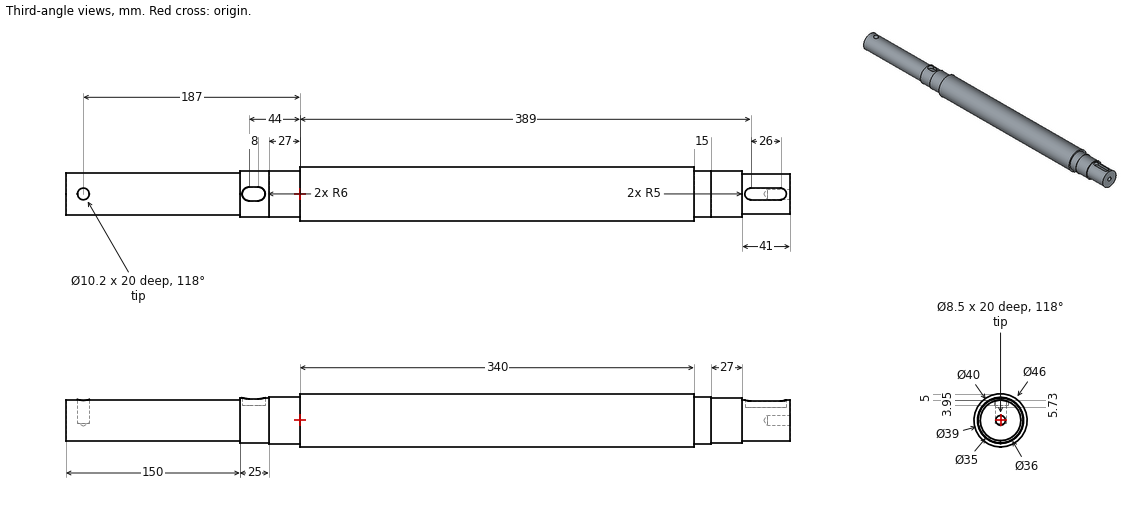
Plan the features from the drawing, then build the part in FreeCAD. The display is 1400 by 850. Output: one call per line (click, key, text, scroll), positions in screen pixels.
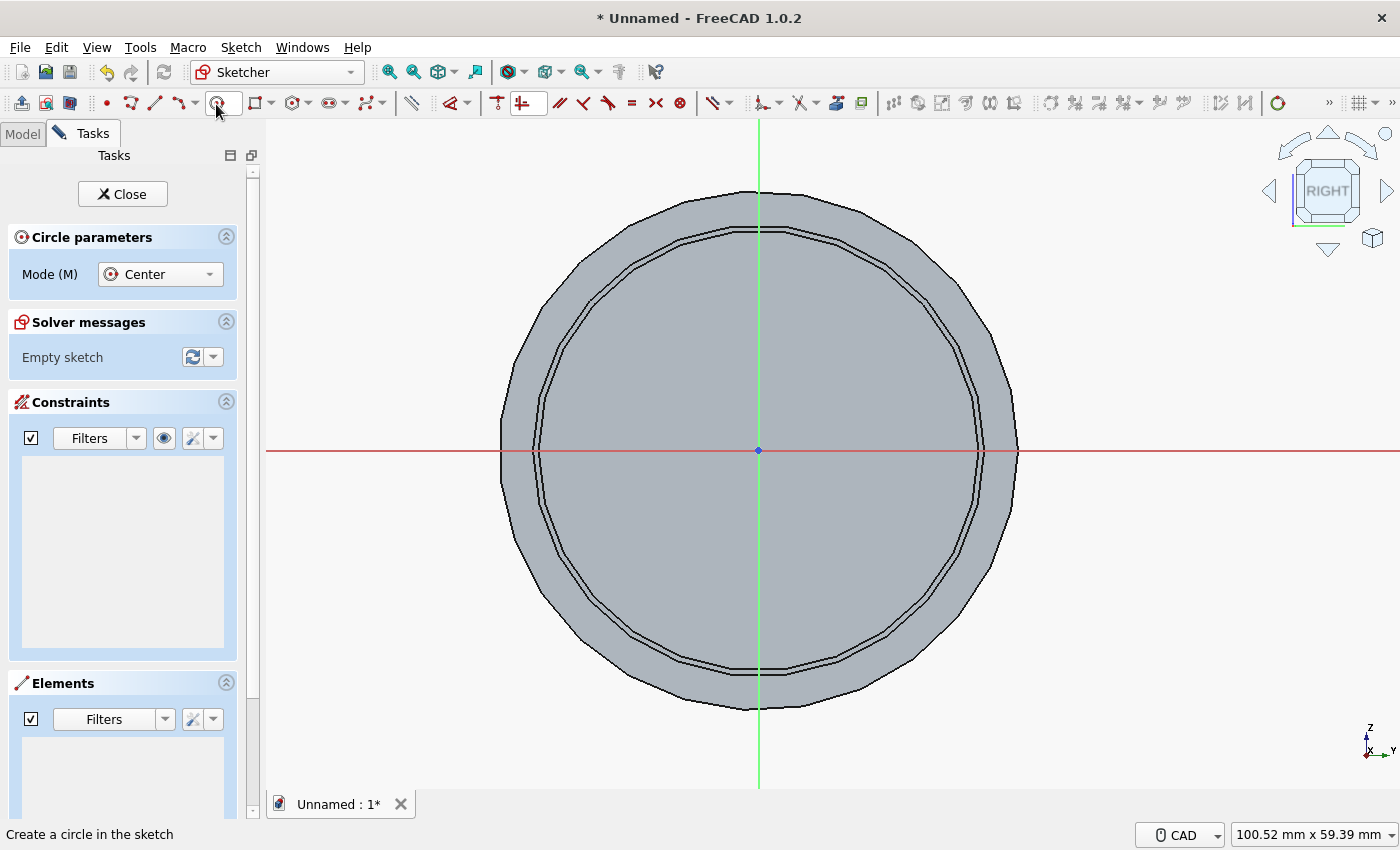
click(759, 451)
click(898, 311)
key(Escape)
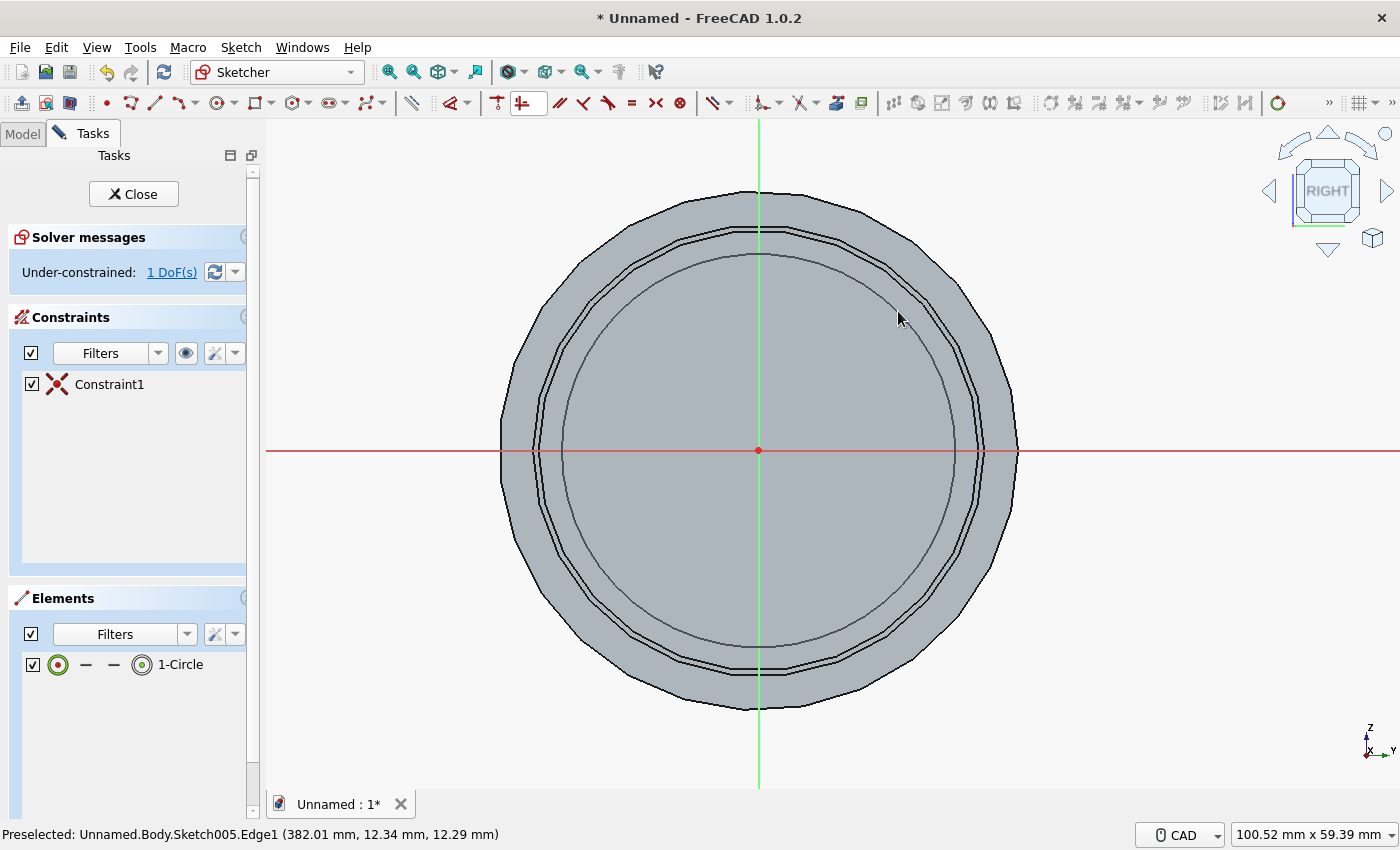
click(450, 104)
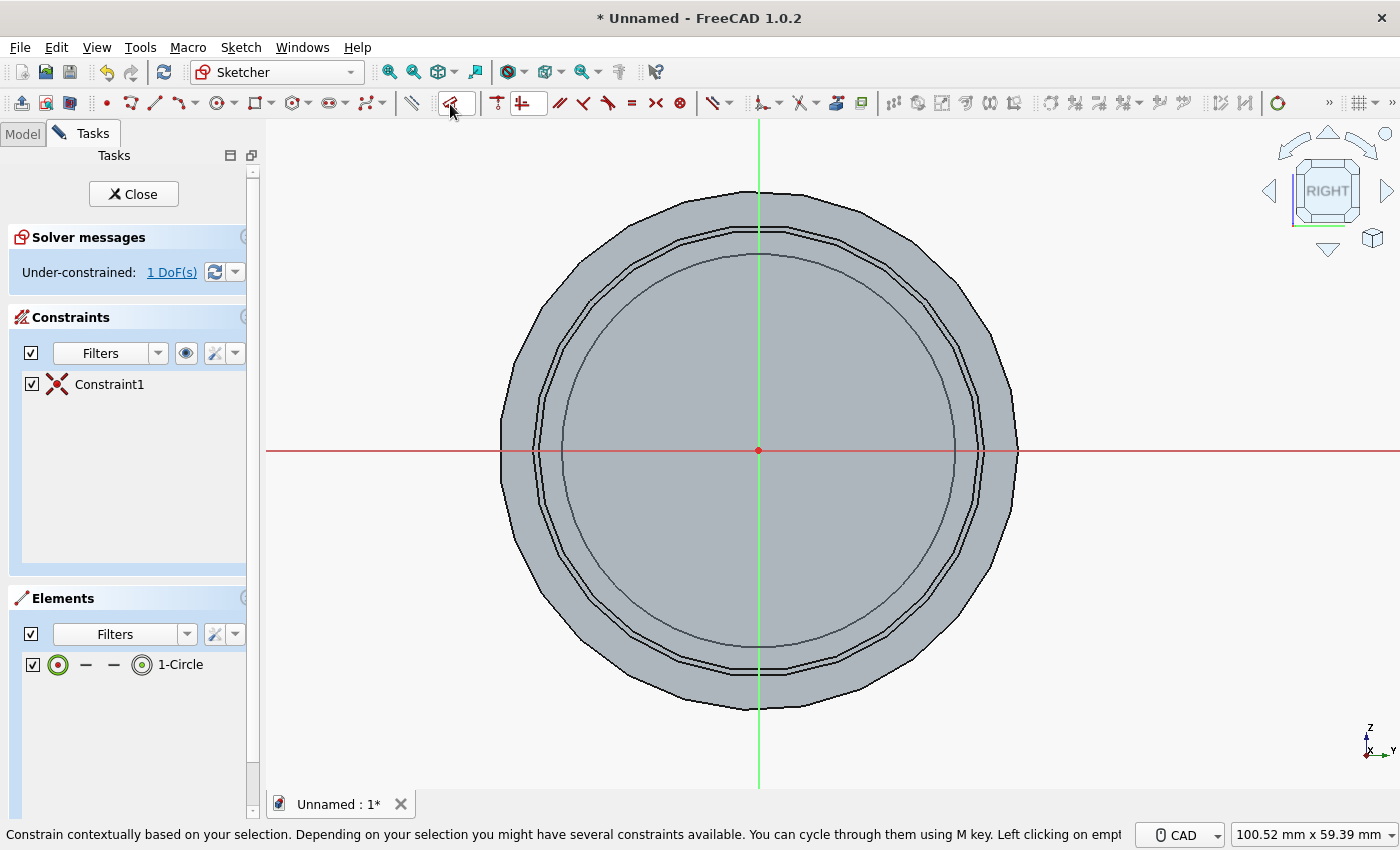
click(897, 311)
click(920, 288)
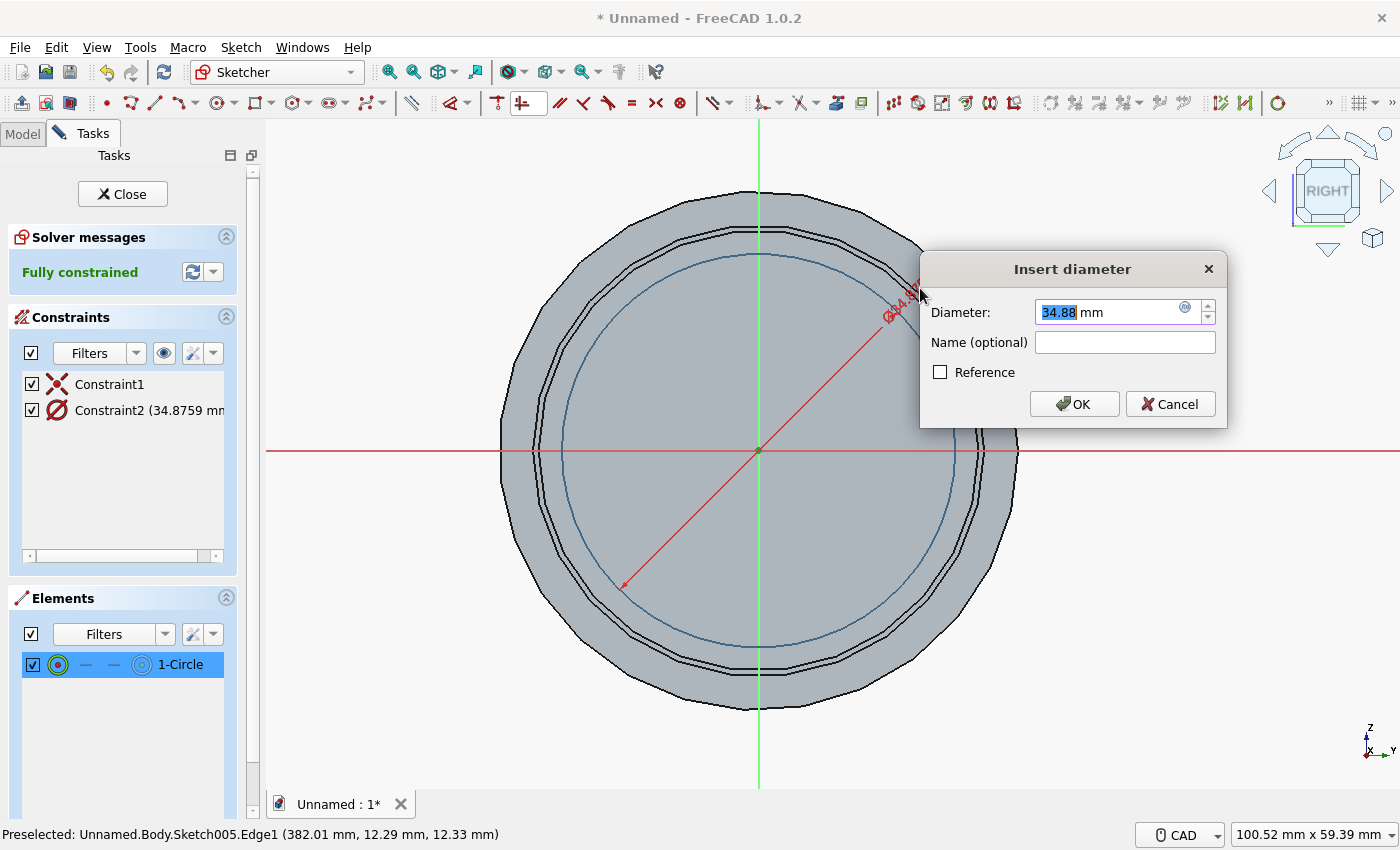
text(35)
key(Return)
key(Escape)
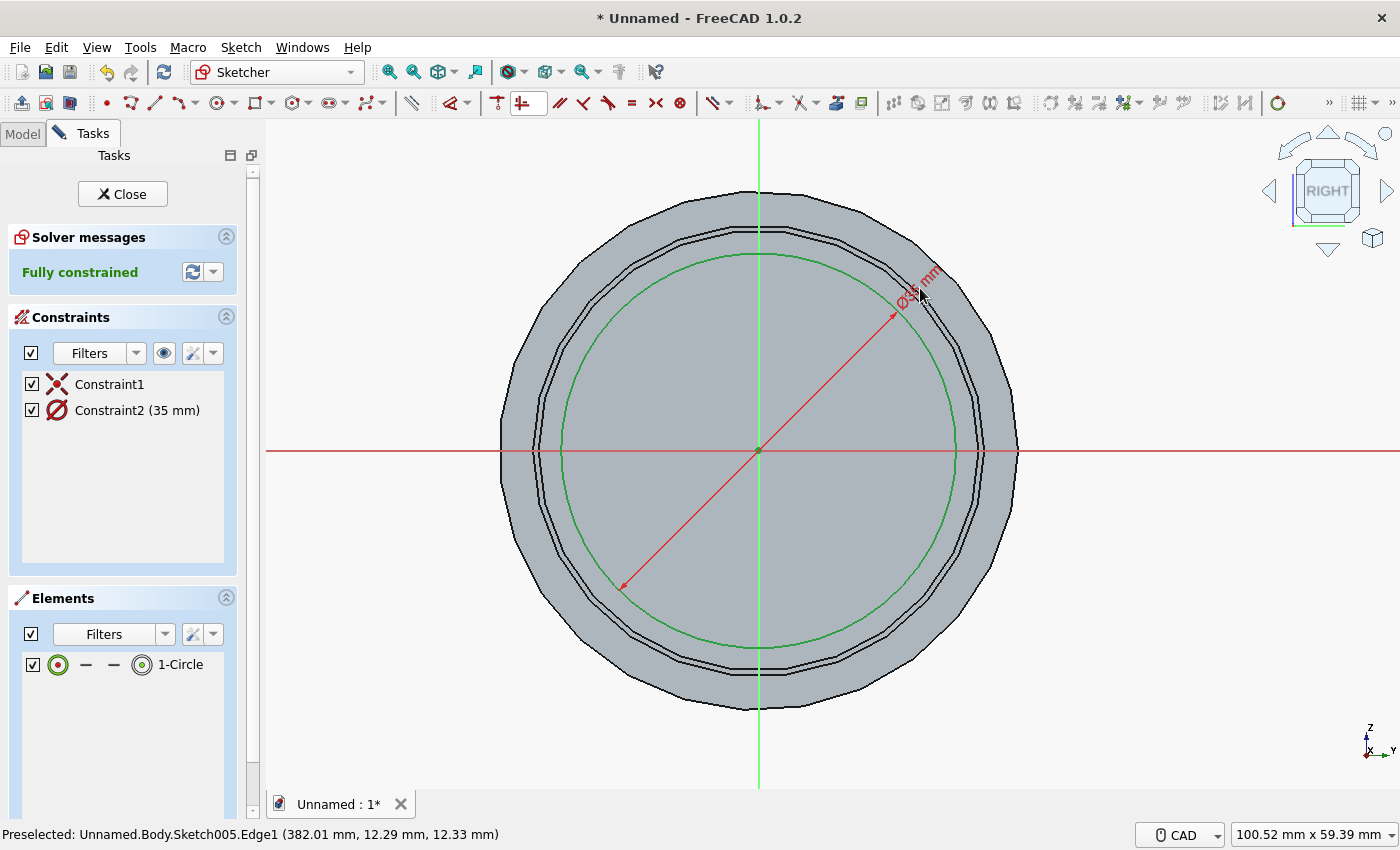
click(123, 194)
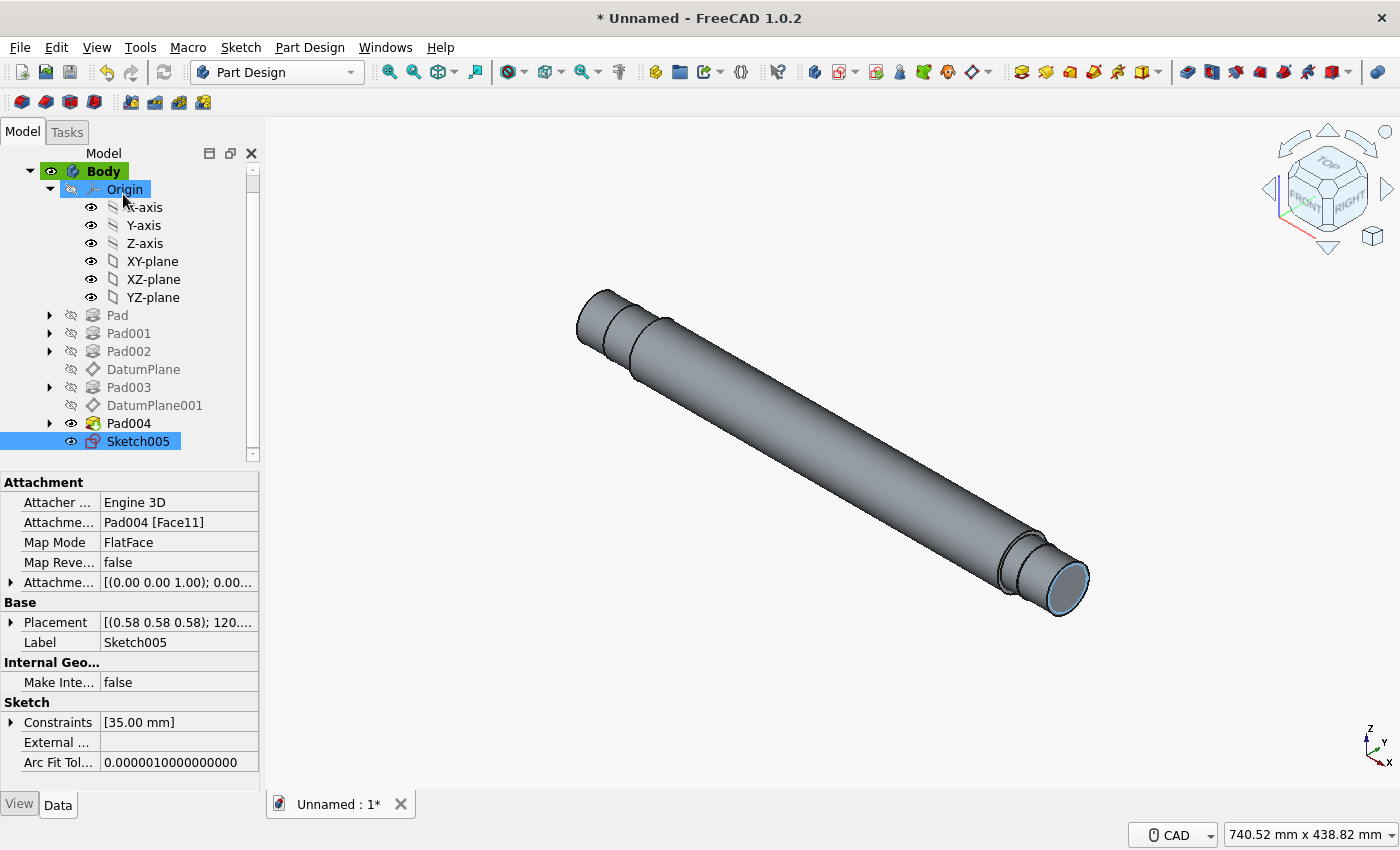
click(1022, 72)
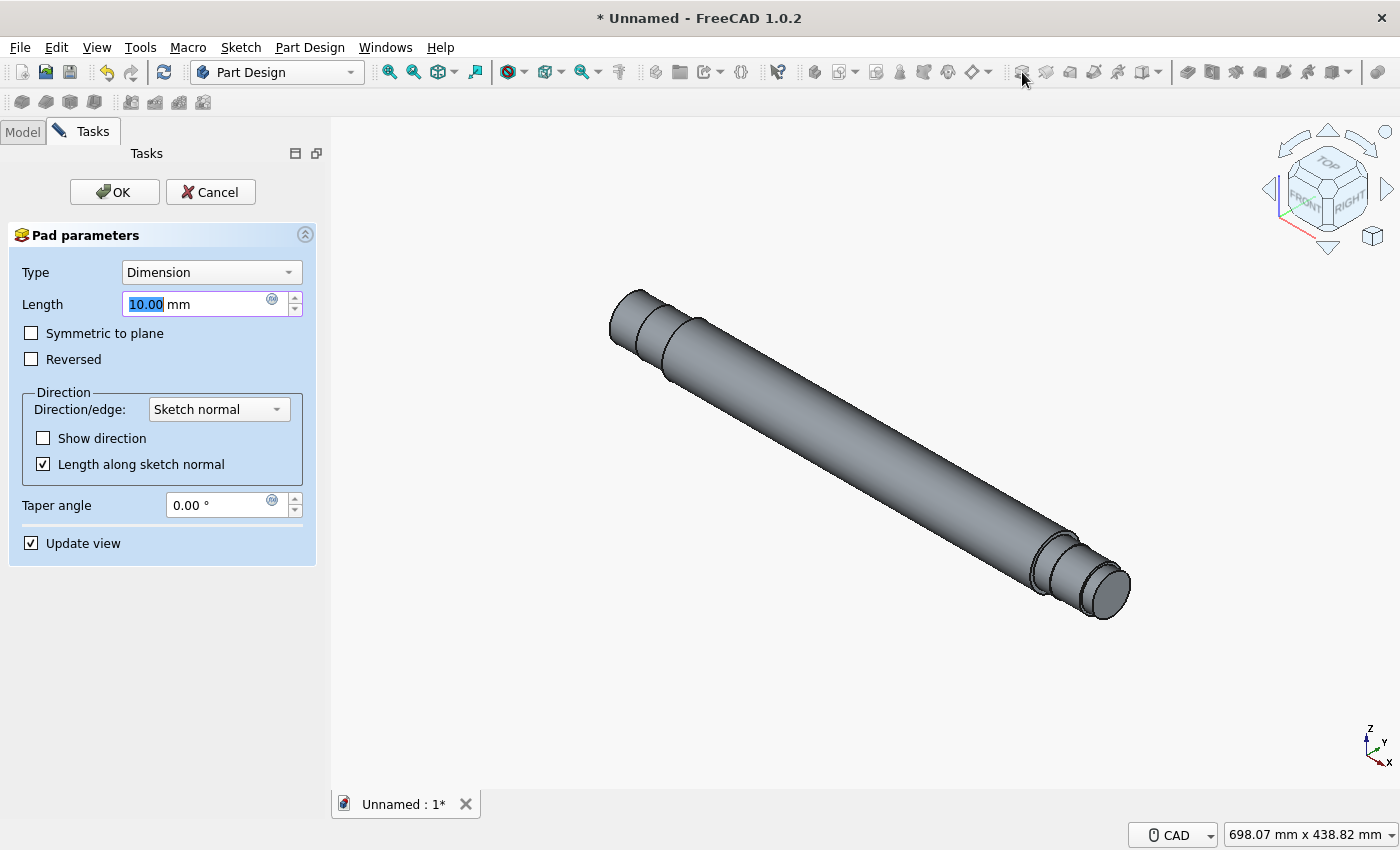
text(41)
key(Tab)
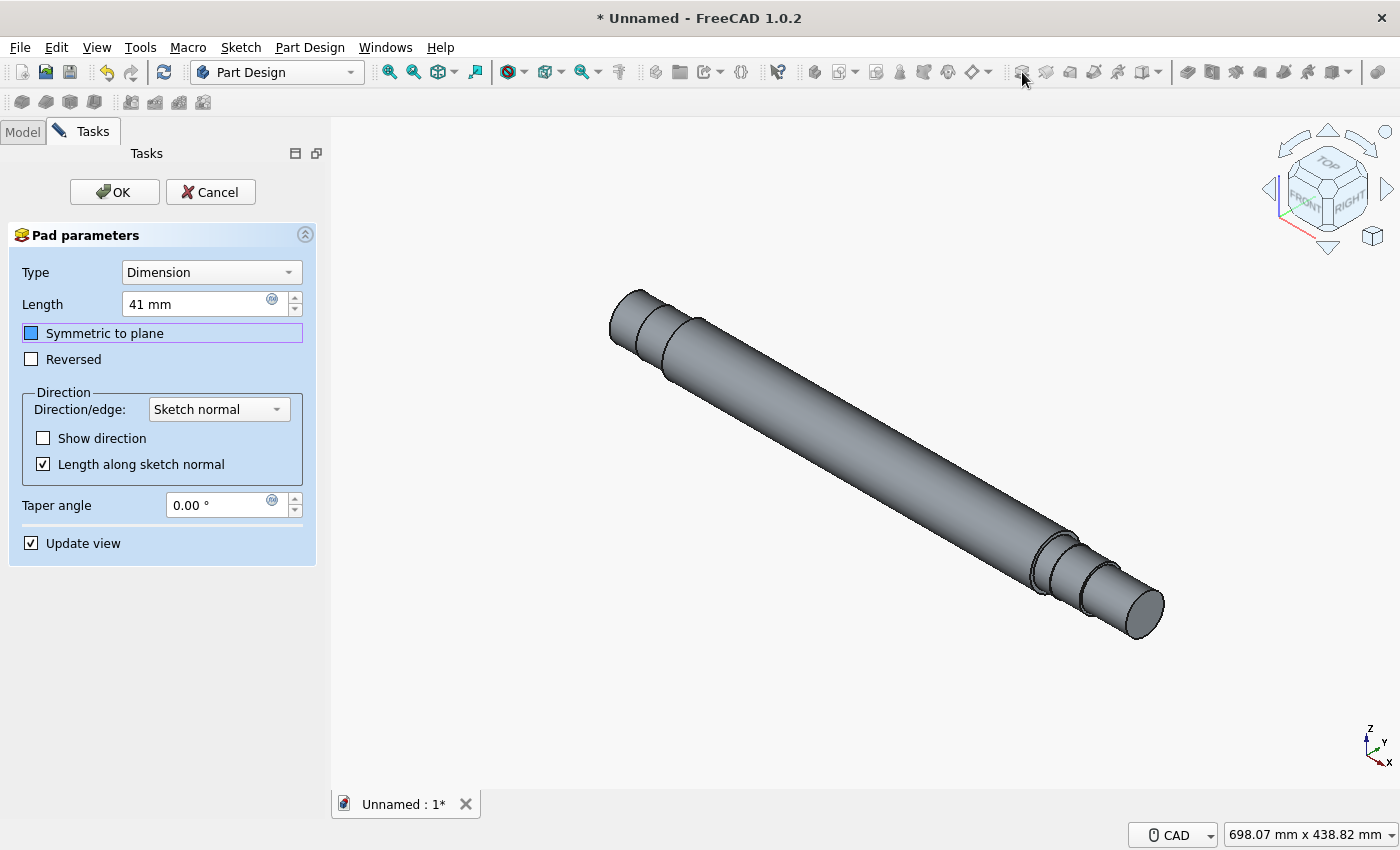
click(115, 192)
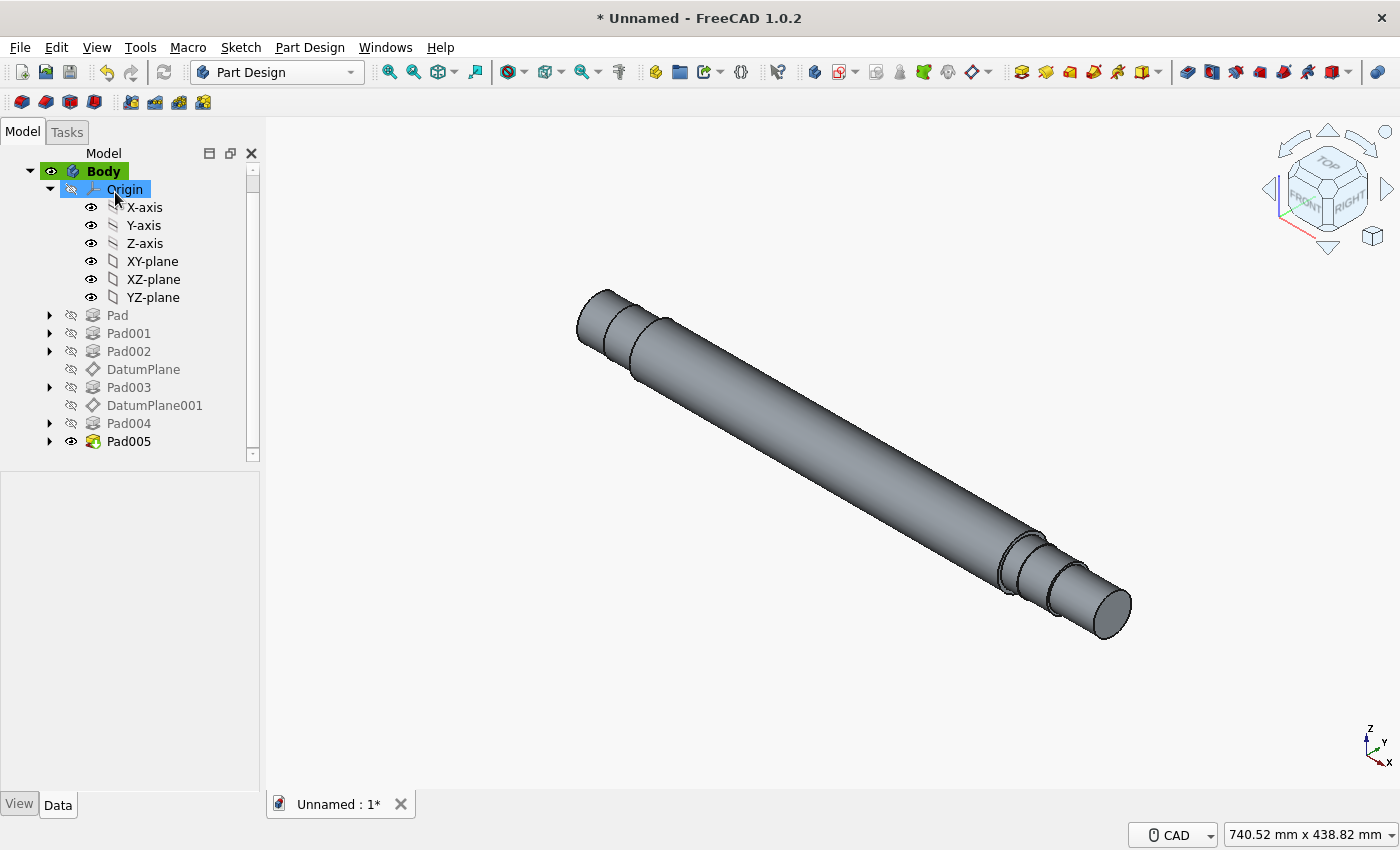
click(136, 261)